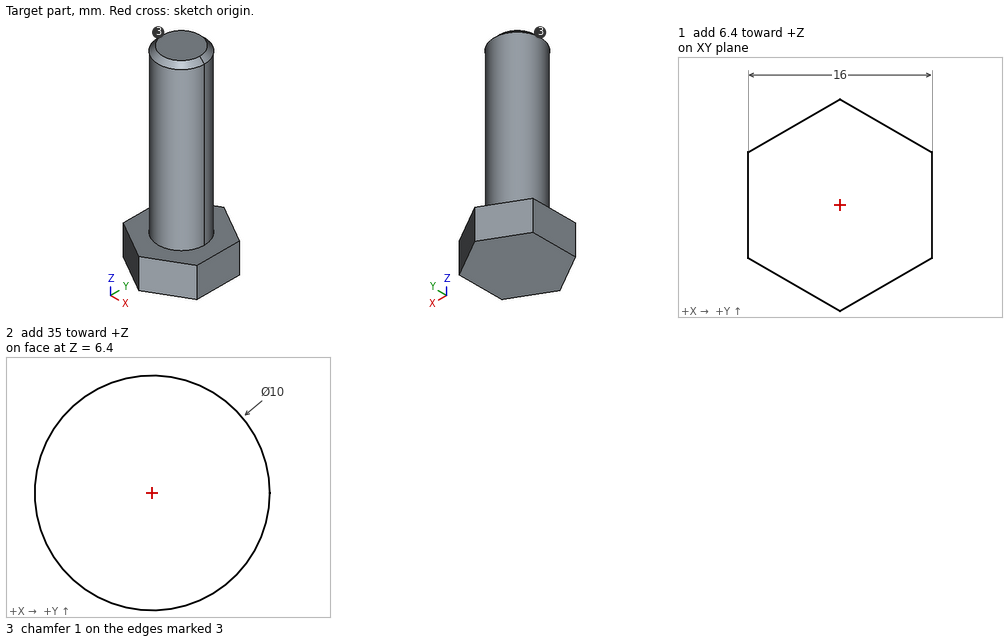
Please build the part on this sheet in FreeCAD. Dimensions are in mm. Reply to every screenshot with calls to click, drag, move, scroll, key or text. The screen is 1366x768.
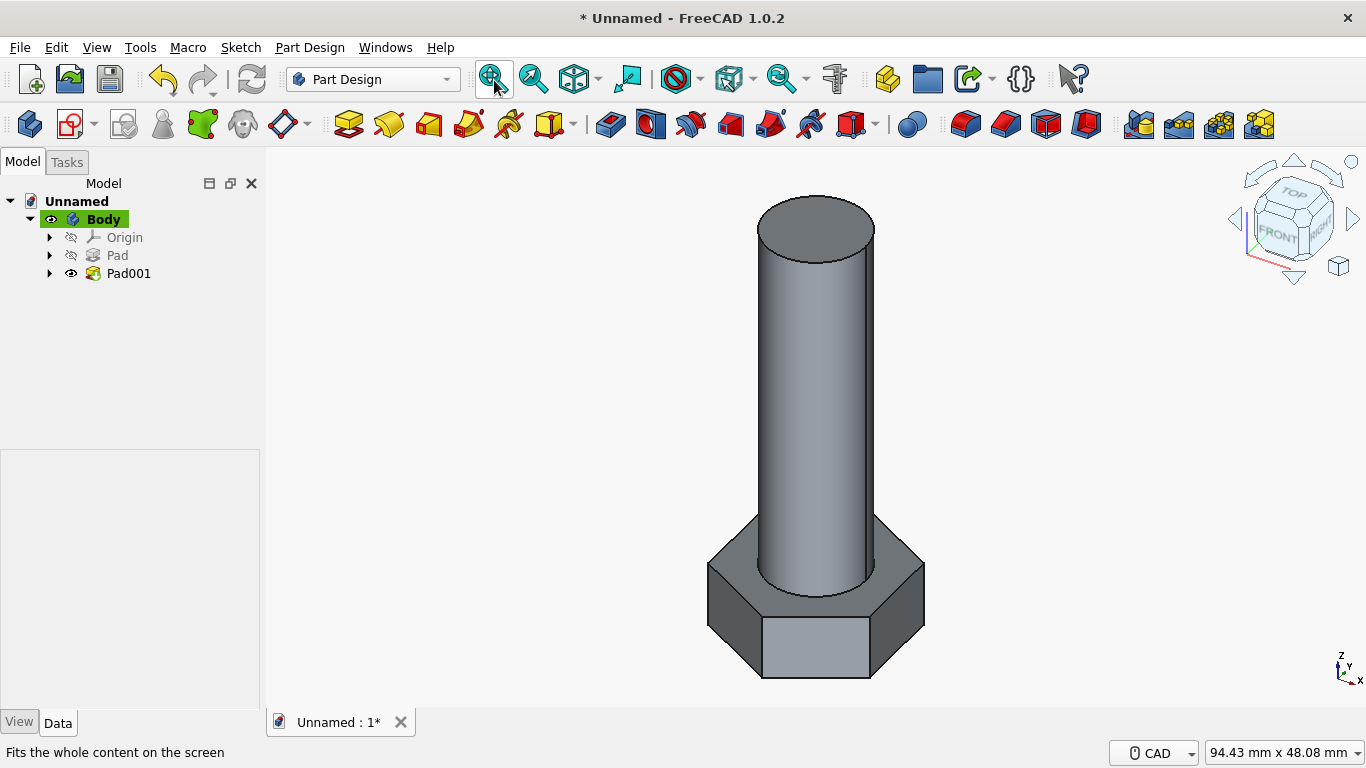
click(758, 232)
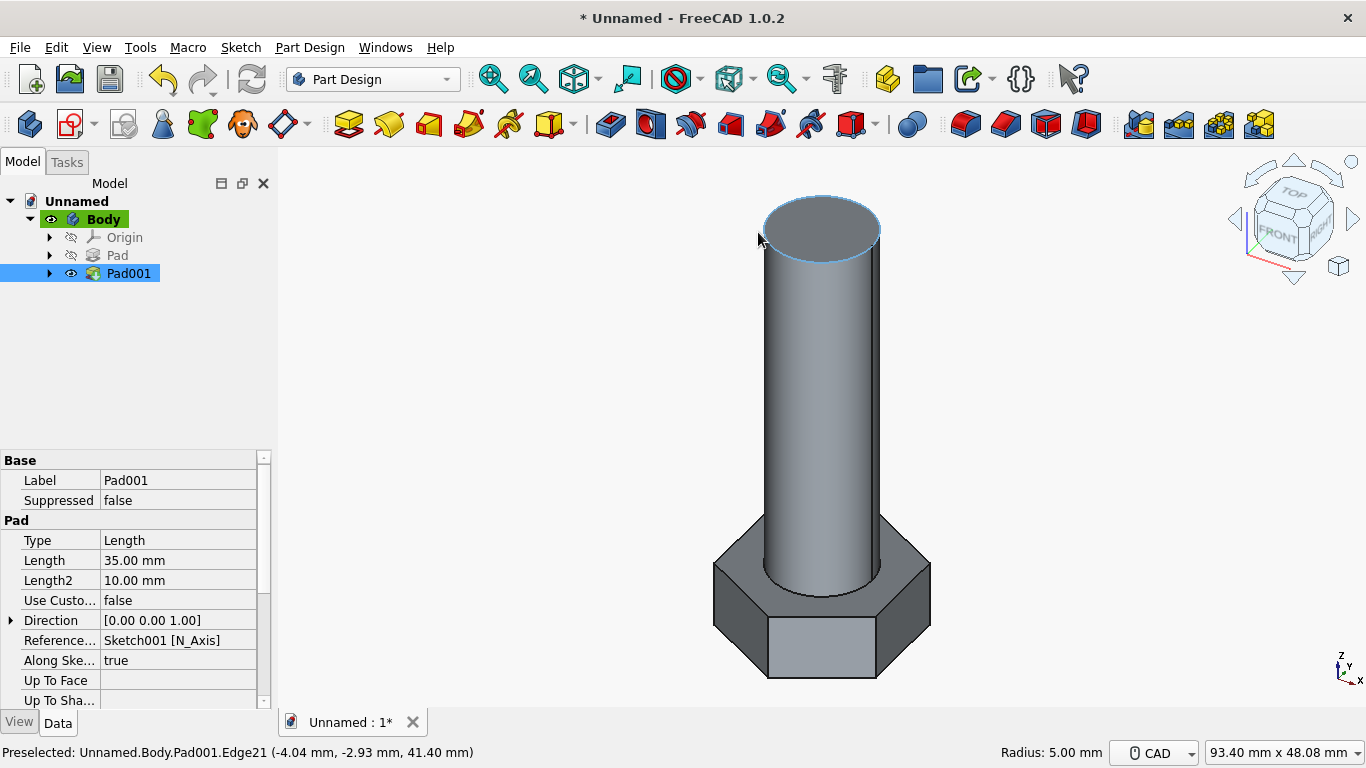
click(1006, 124)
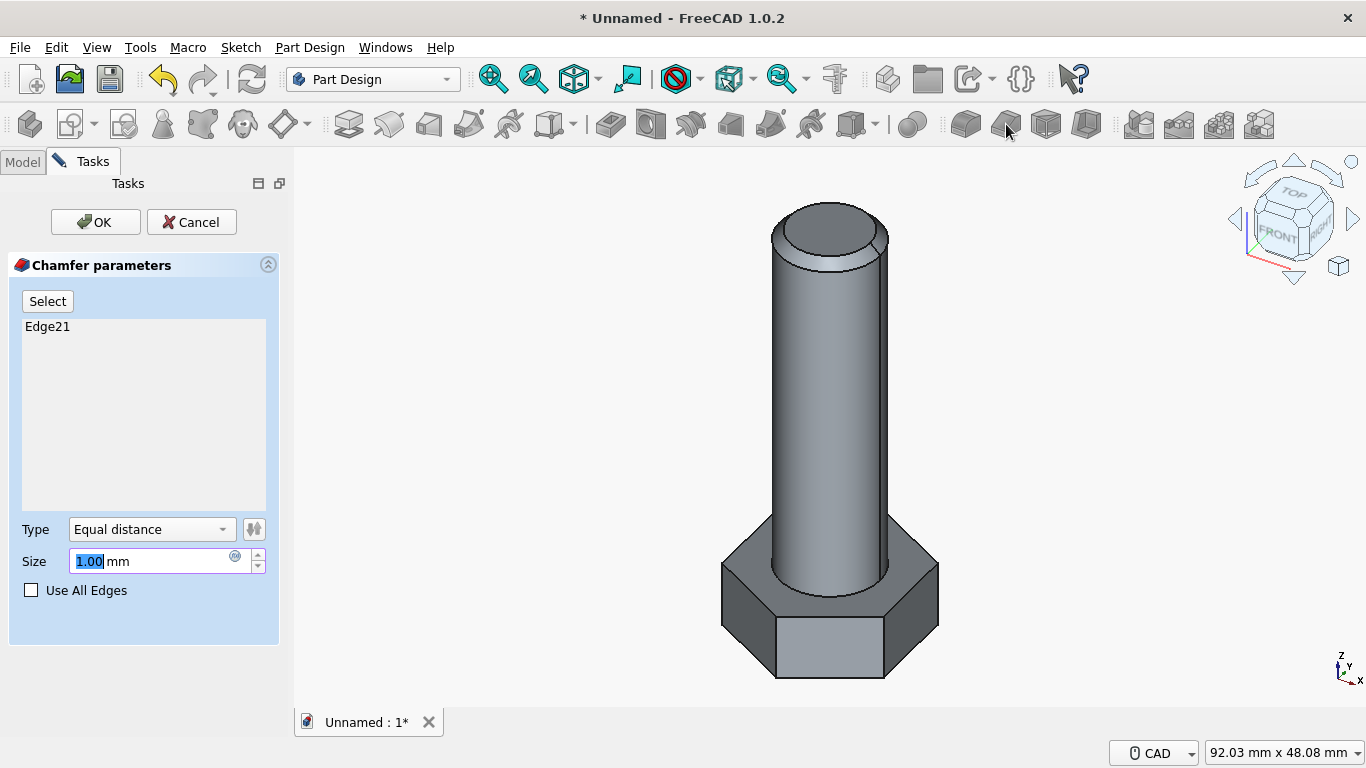
text(1)
key(Tab)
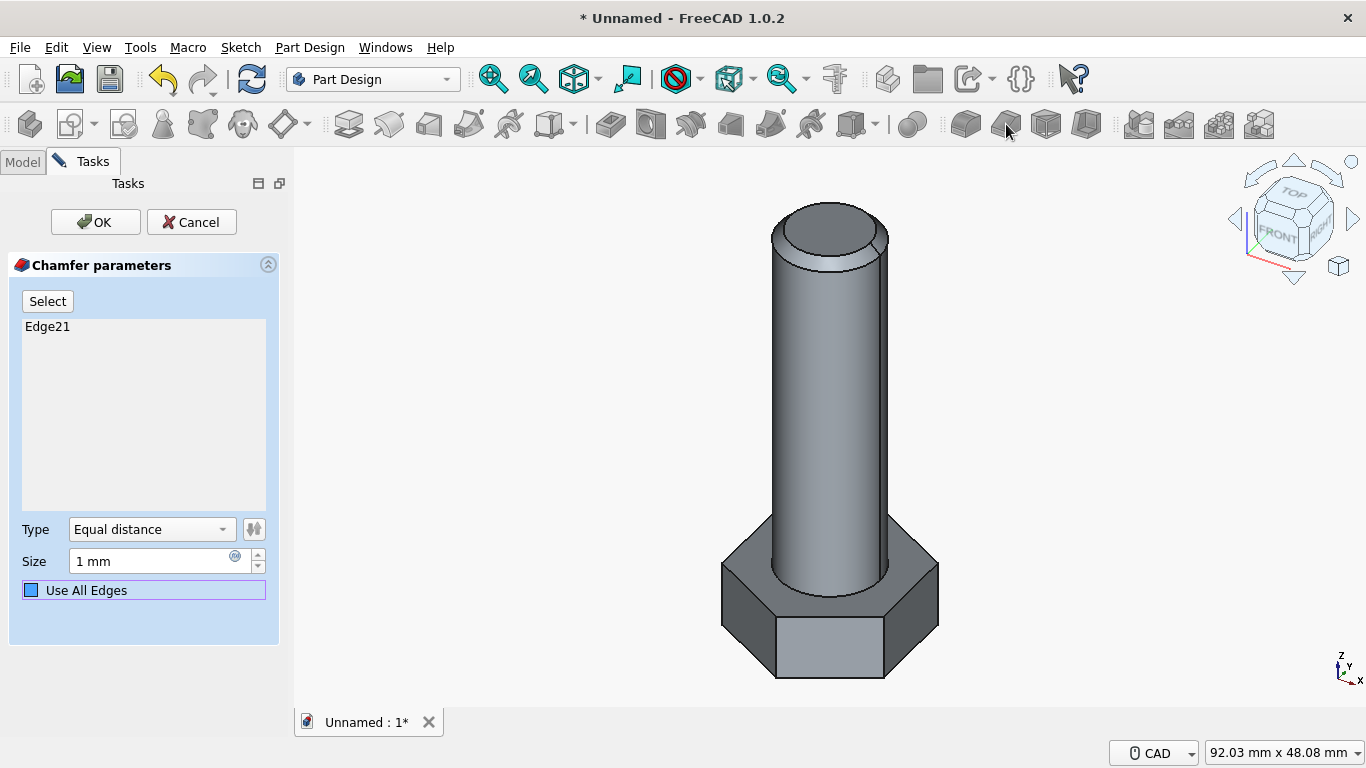
click(96, 222)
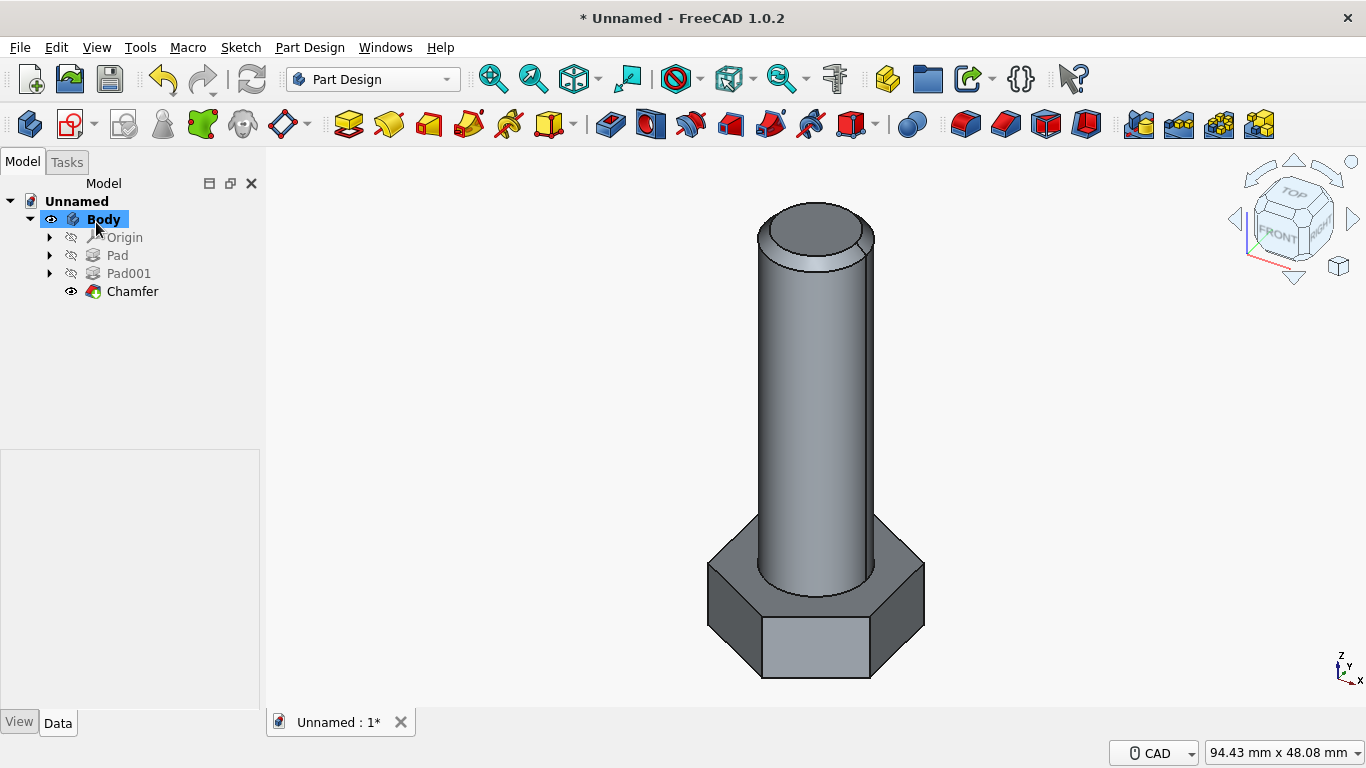
key(0)